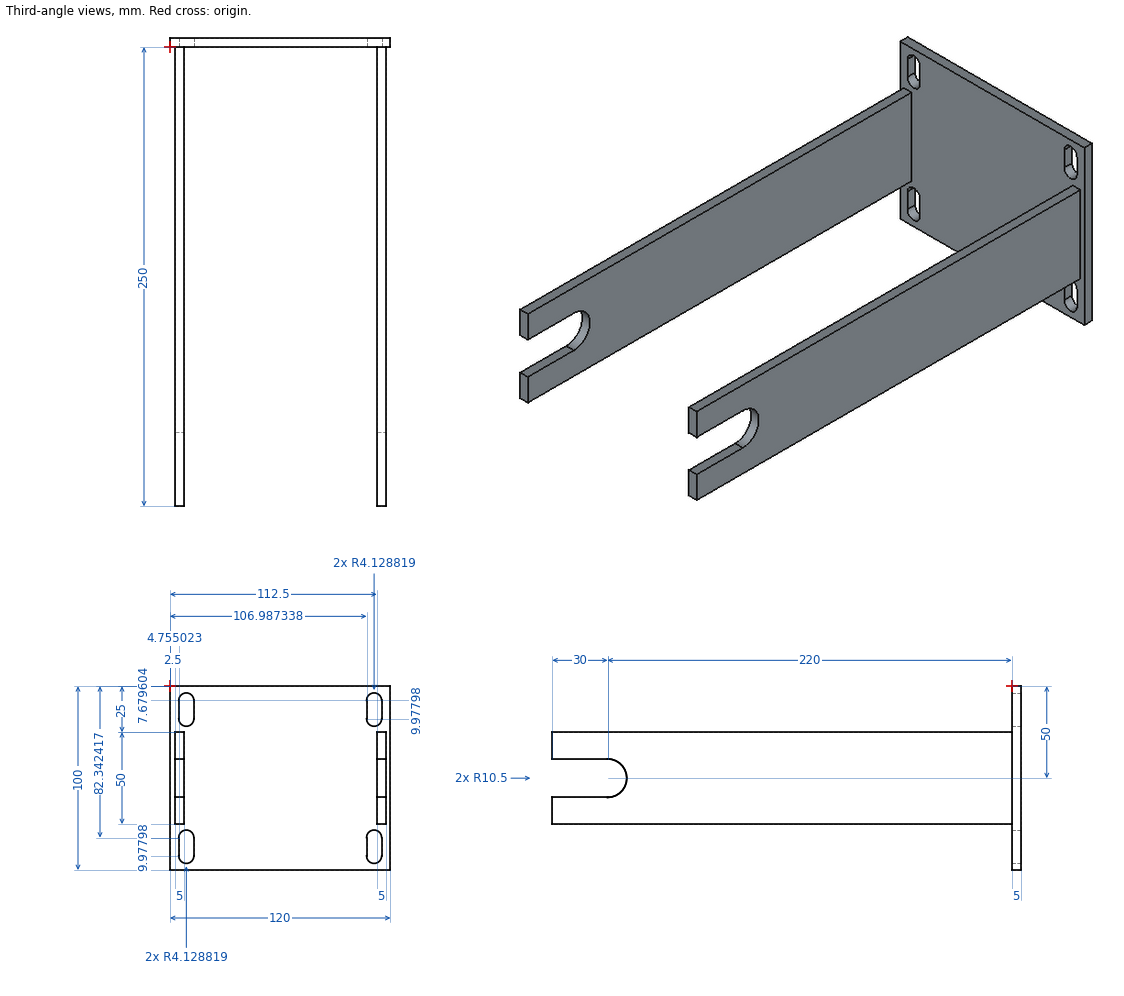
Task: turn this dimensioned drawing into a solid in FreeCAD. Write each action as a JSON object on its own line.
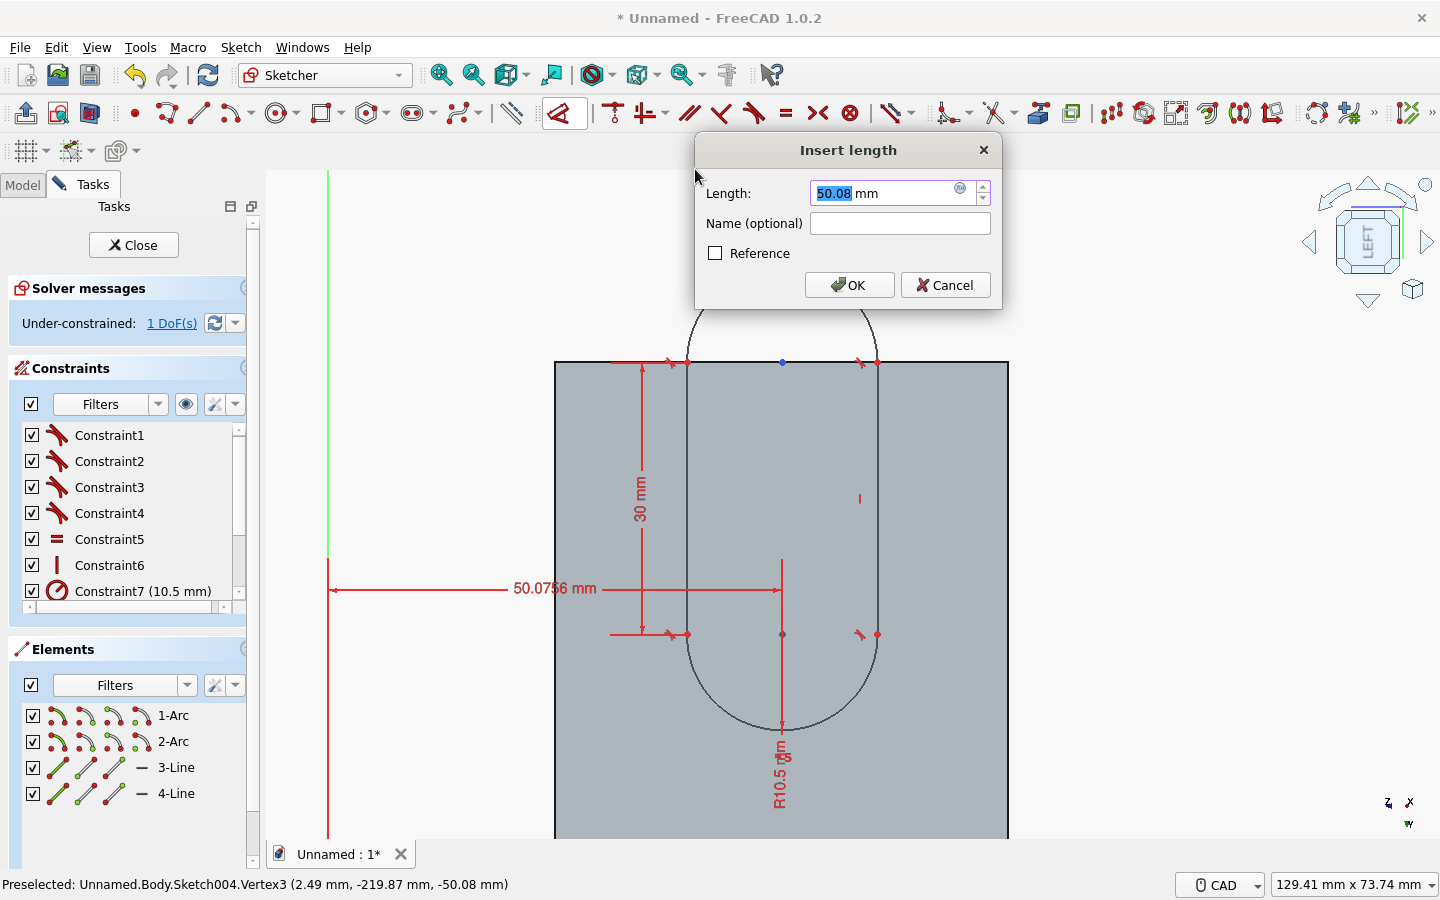
{"action": "type", "text": "50"}
{"action": "key", "text": "Return"}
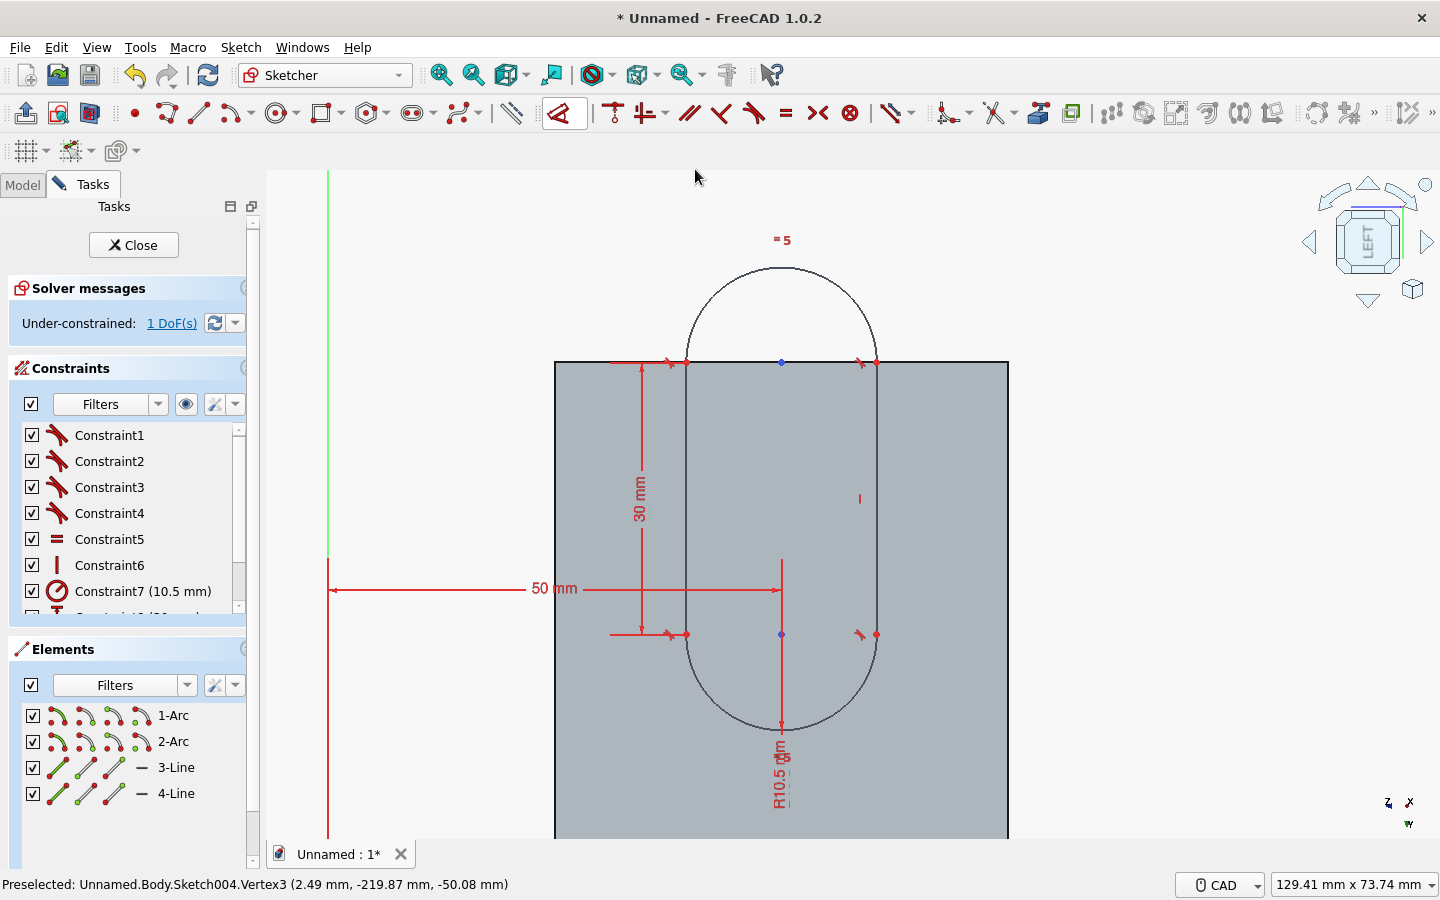
{"action": "left_click", "coordinate": [686, 635]}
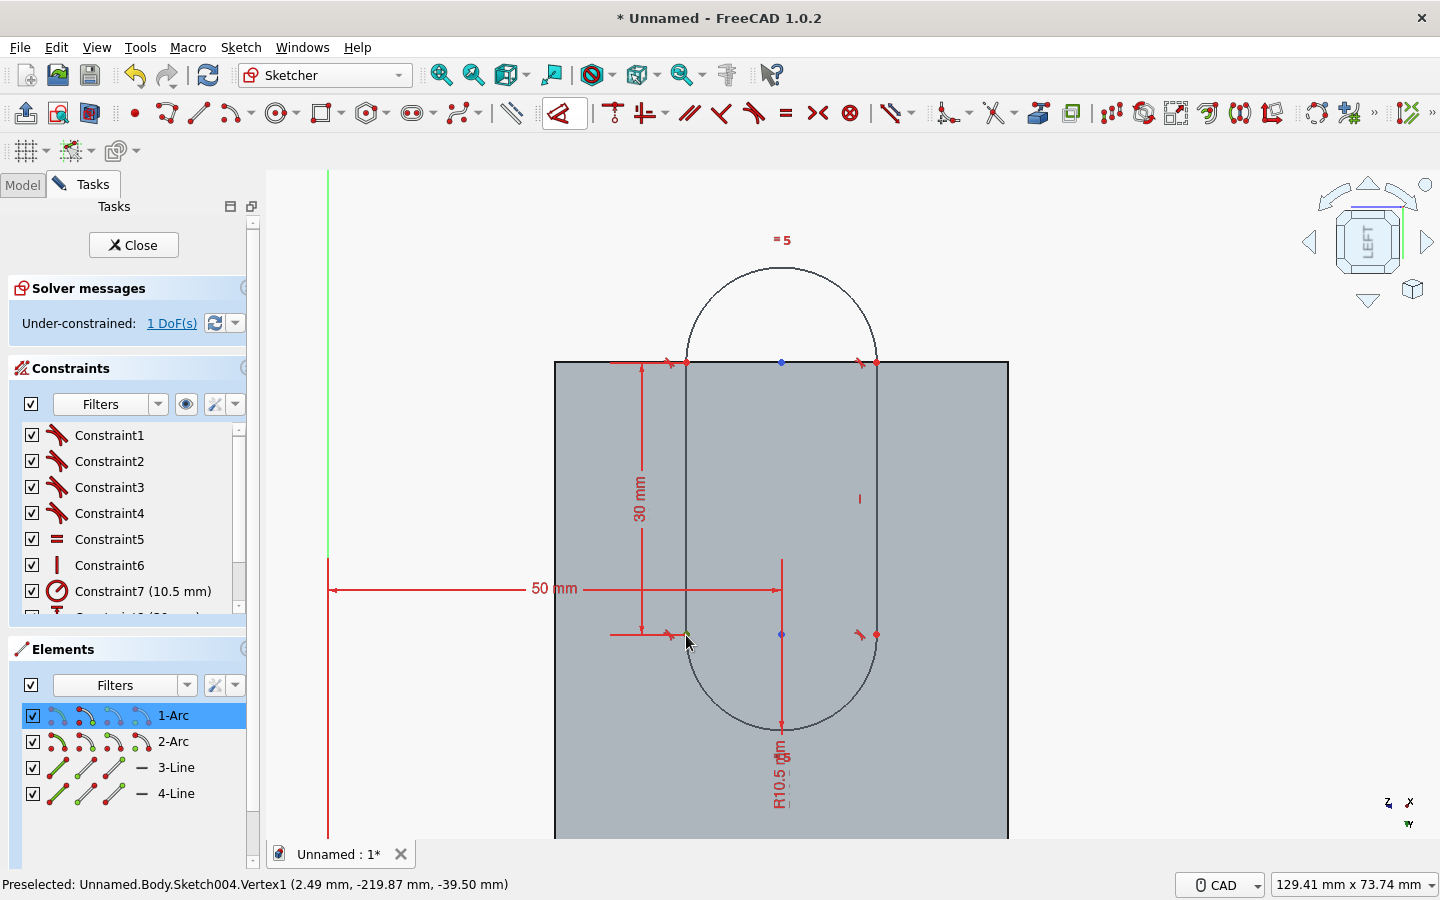
{"action": "key", "text": "i"}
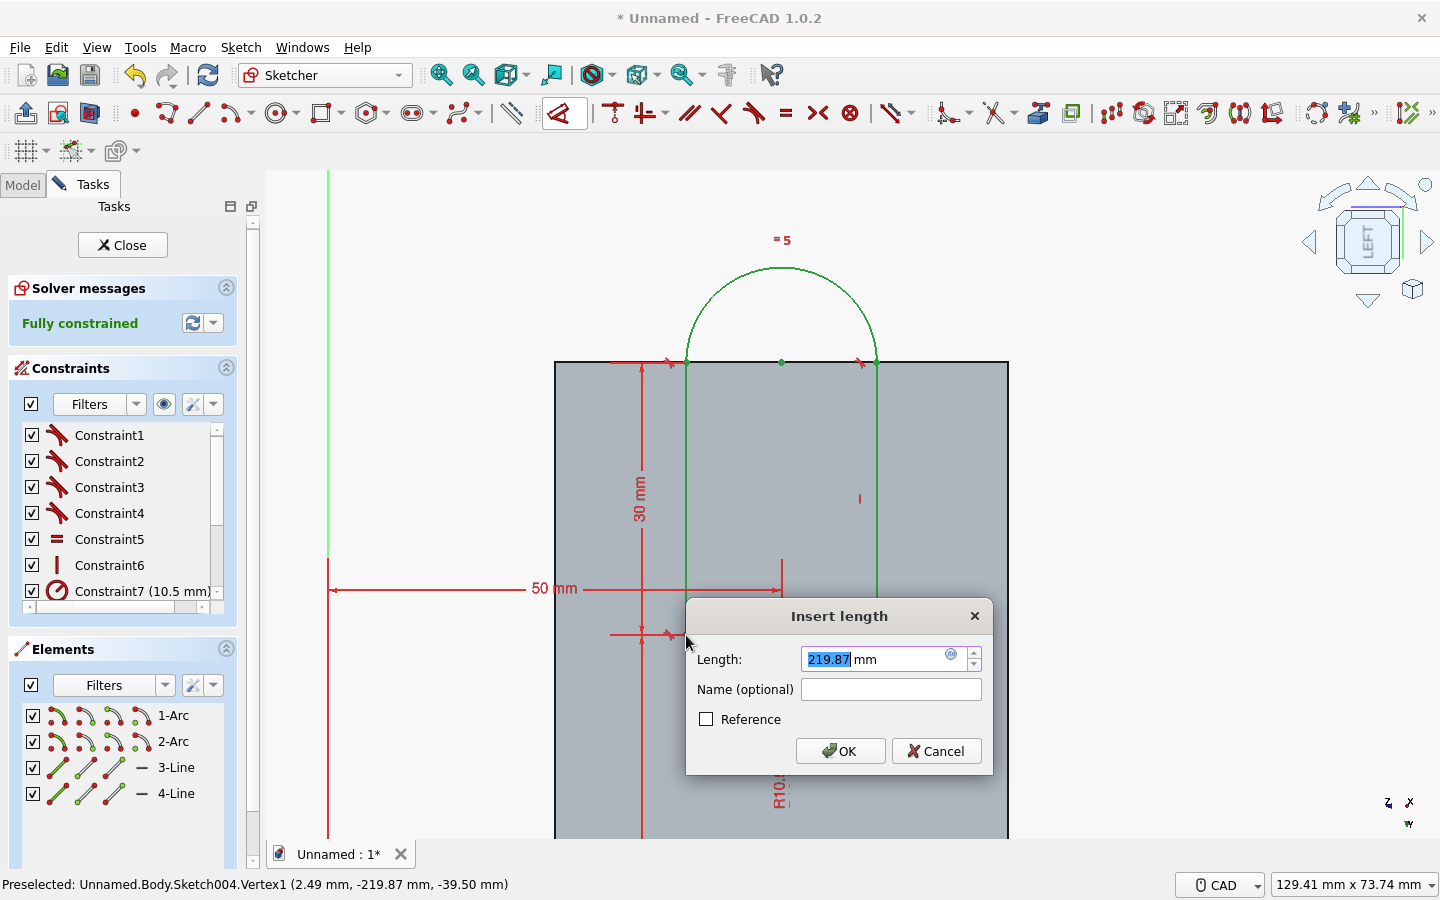
{"action": "type", "text": "220"}
{"action": "key", "text": "Return"}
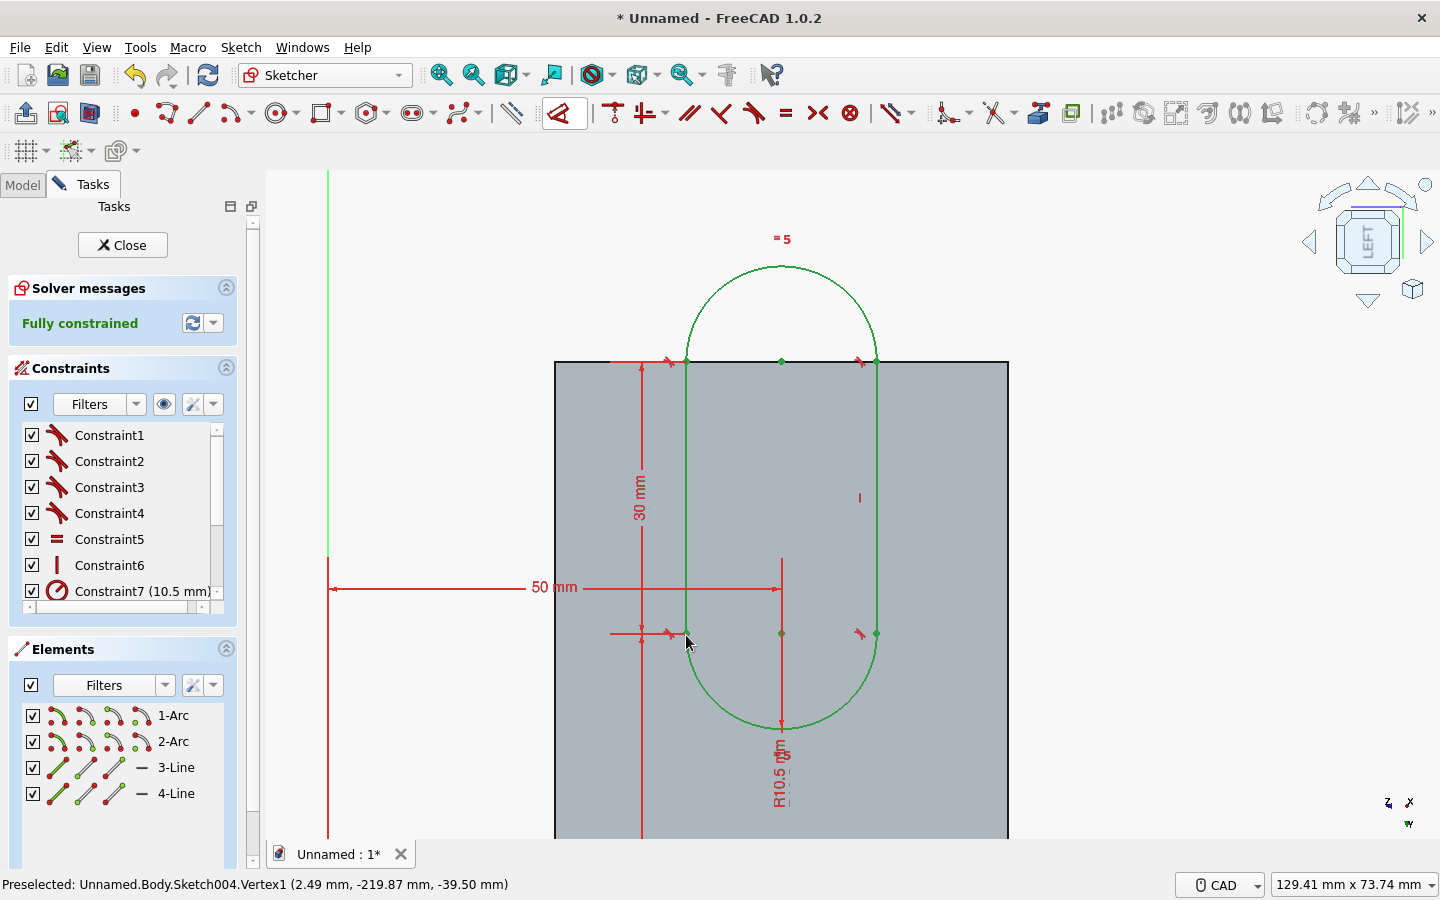
{"action": "left_click", "coordinate": [123, 245]}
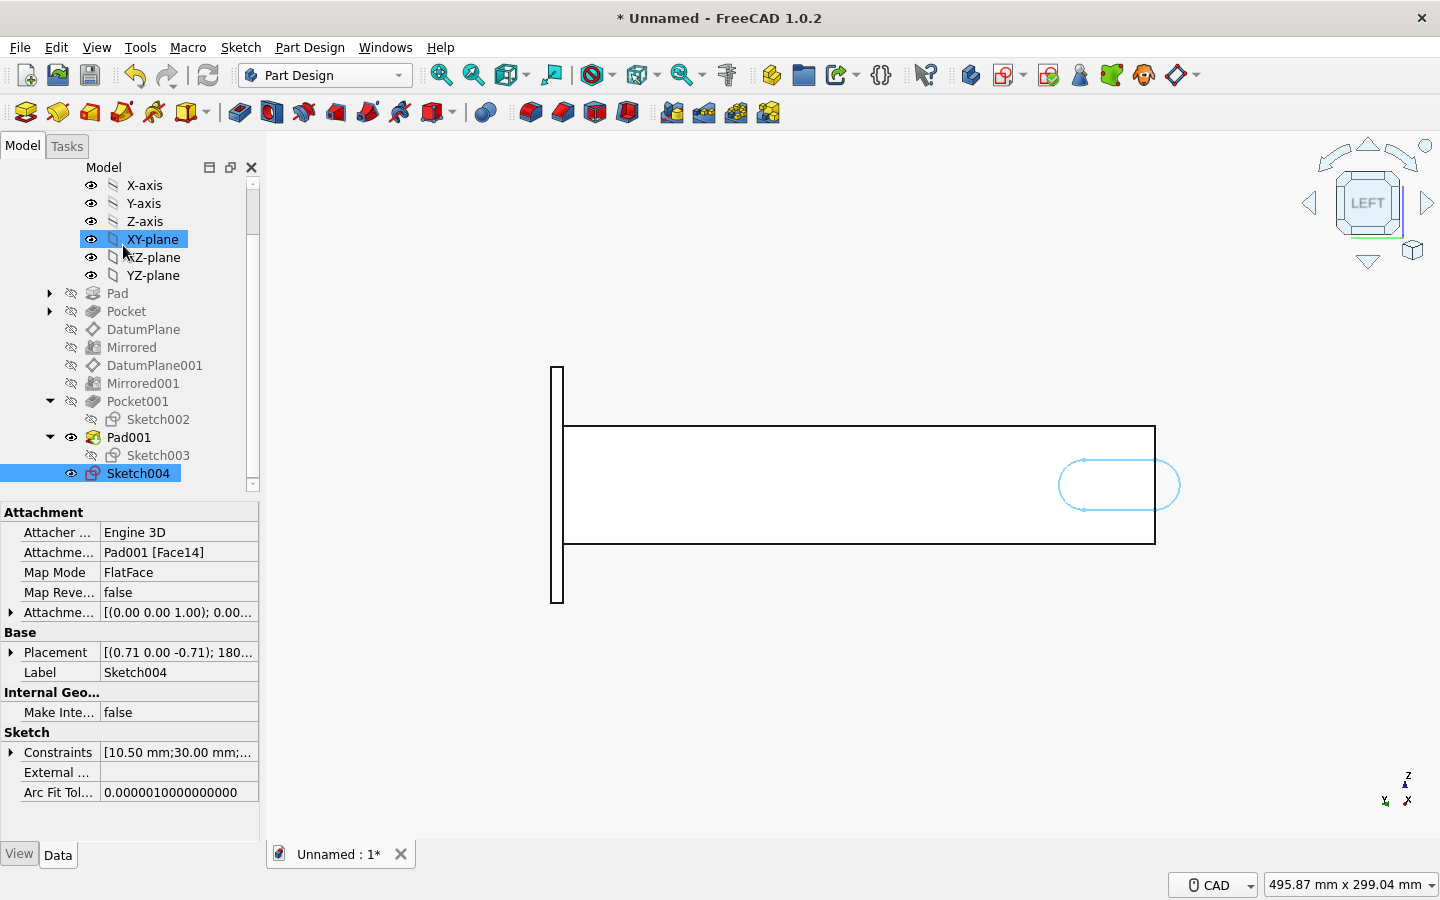
{"action": "left_click", "coordinate": [240, 112]}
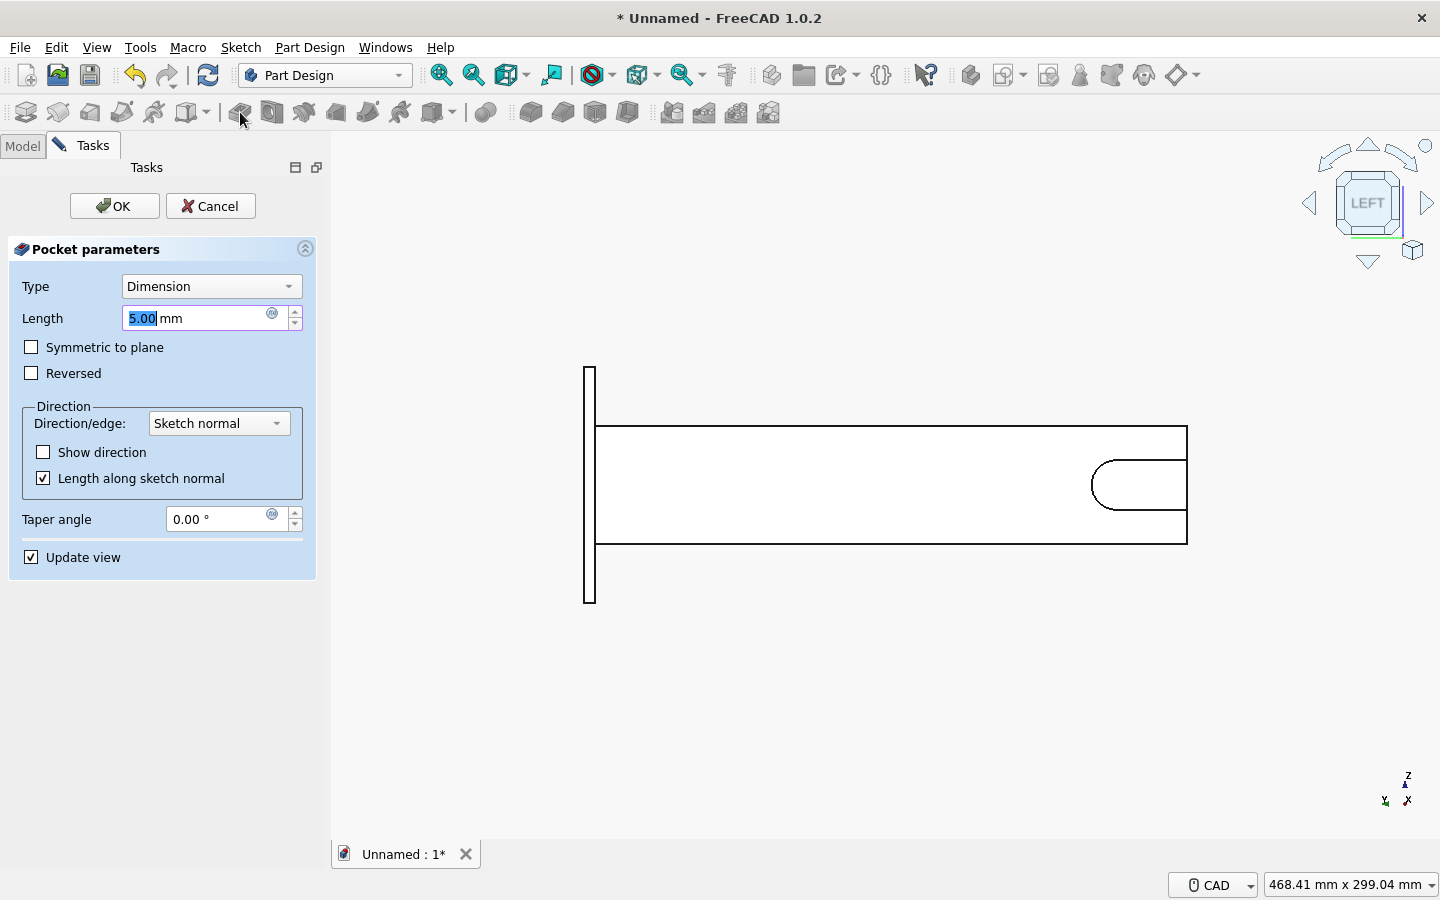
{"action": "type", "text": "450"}
{"action": "key", "text": "Tab"}